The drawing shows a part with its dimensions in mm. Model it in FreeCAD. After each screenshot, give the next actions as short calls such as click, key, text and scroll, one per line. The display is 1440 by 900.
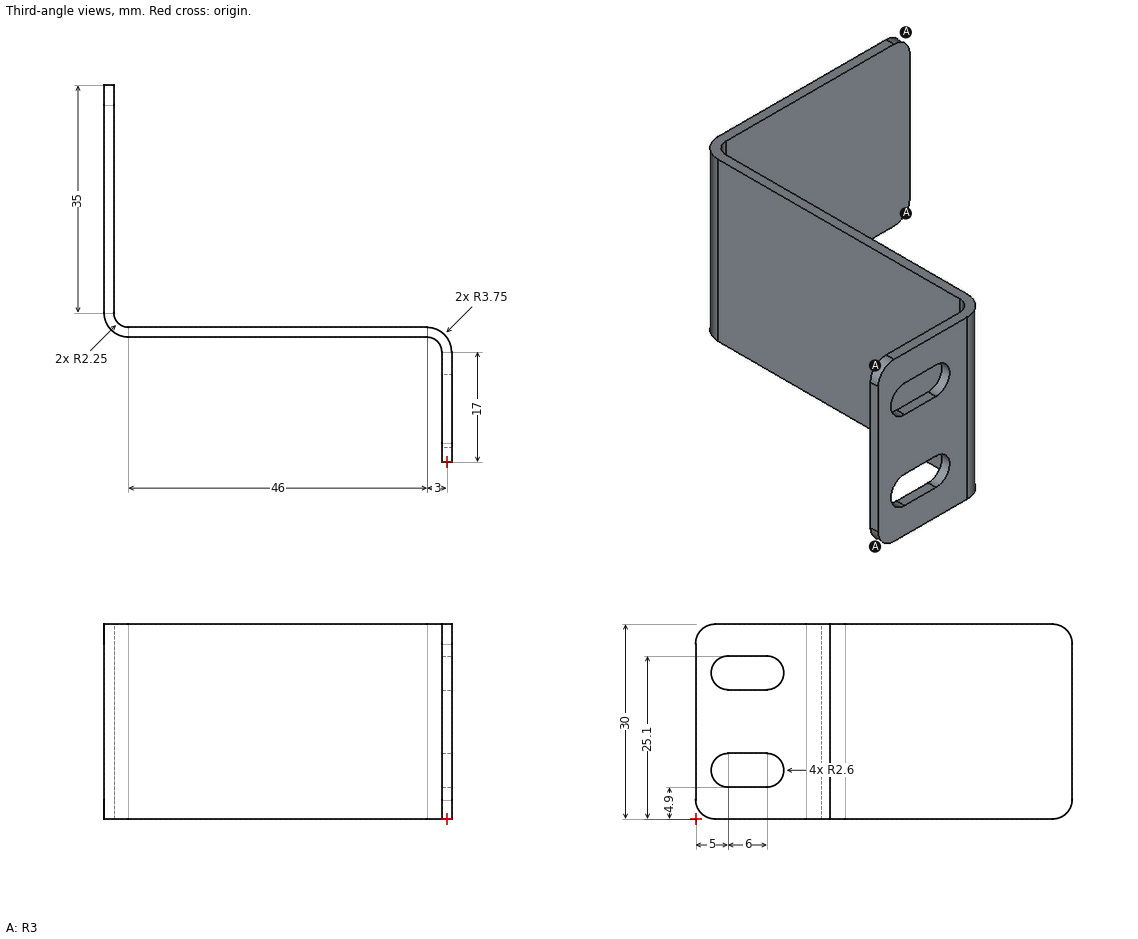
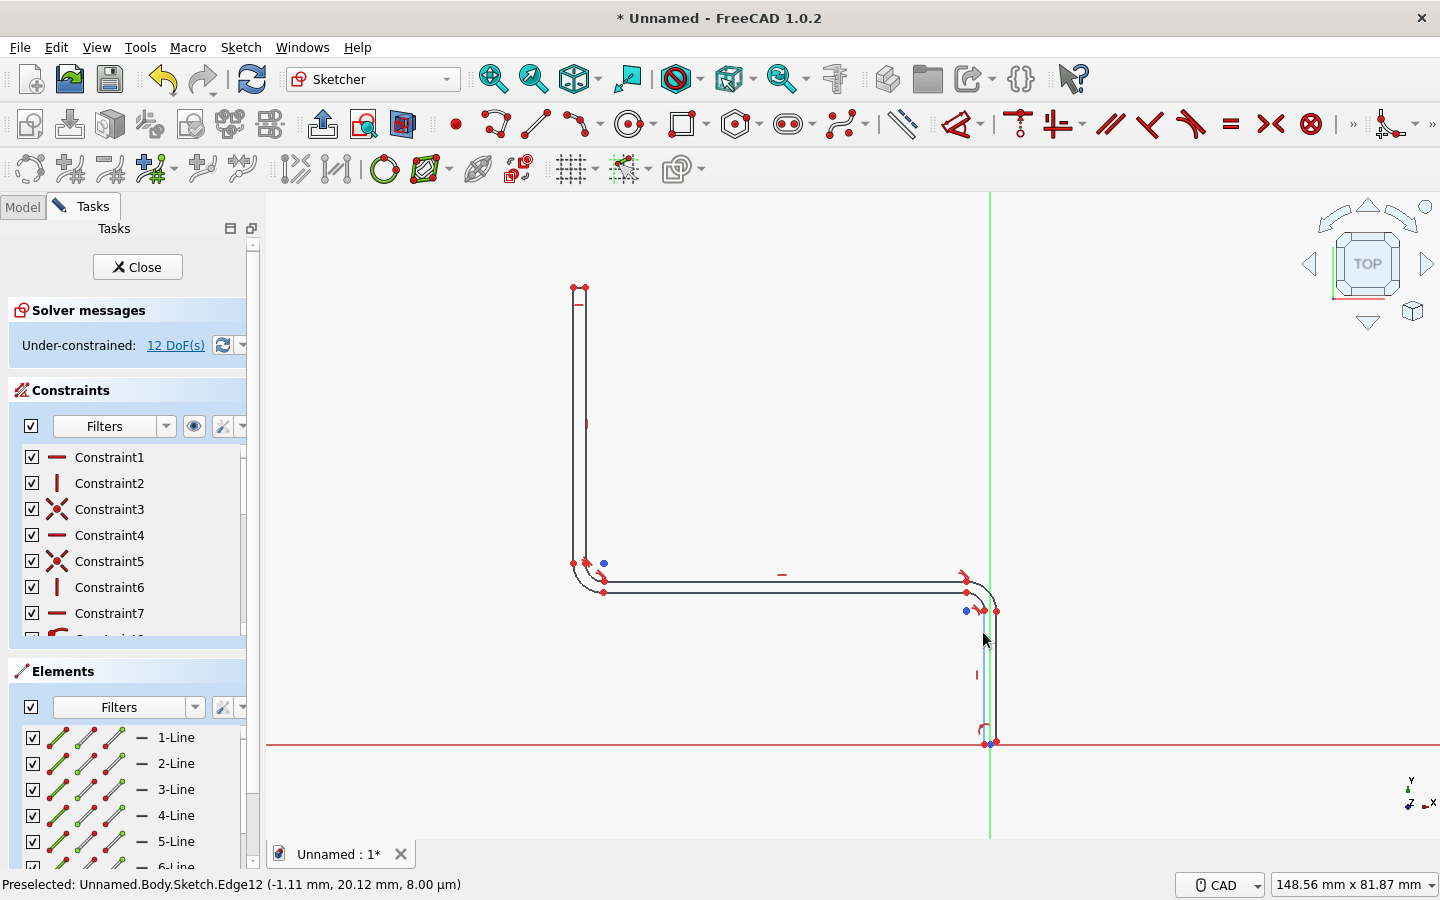
scroll(989, 744, up, 6)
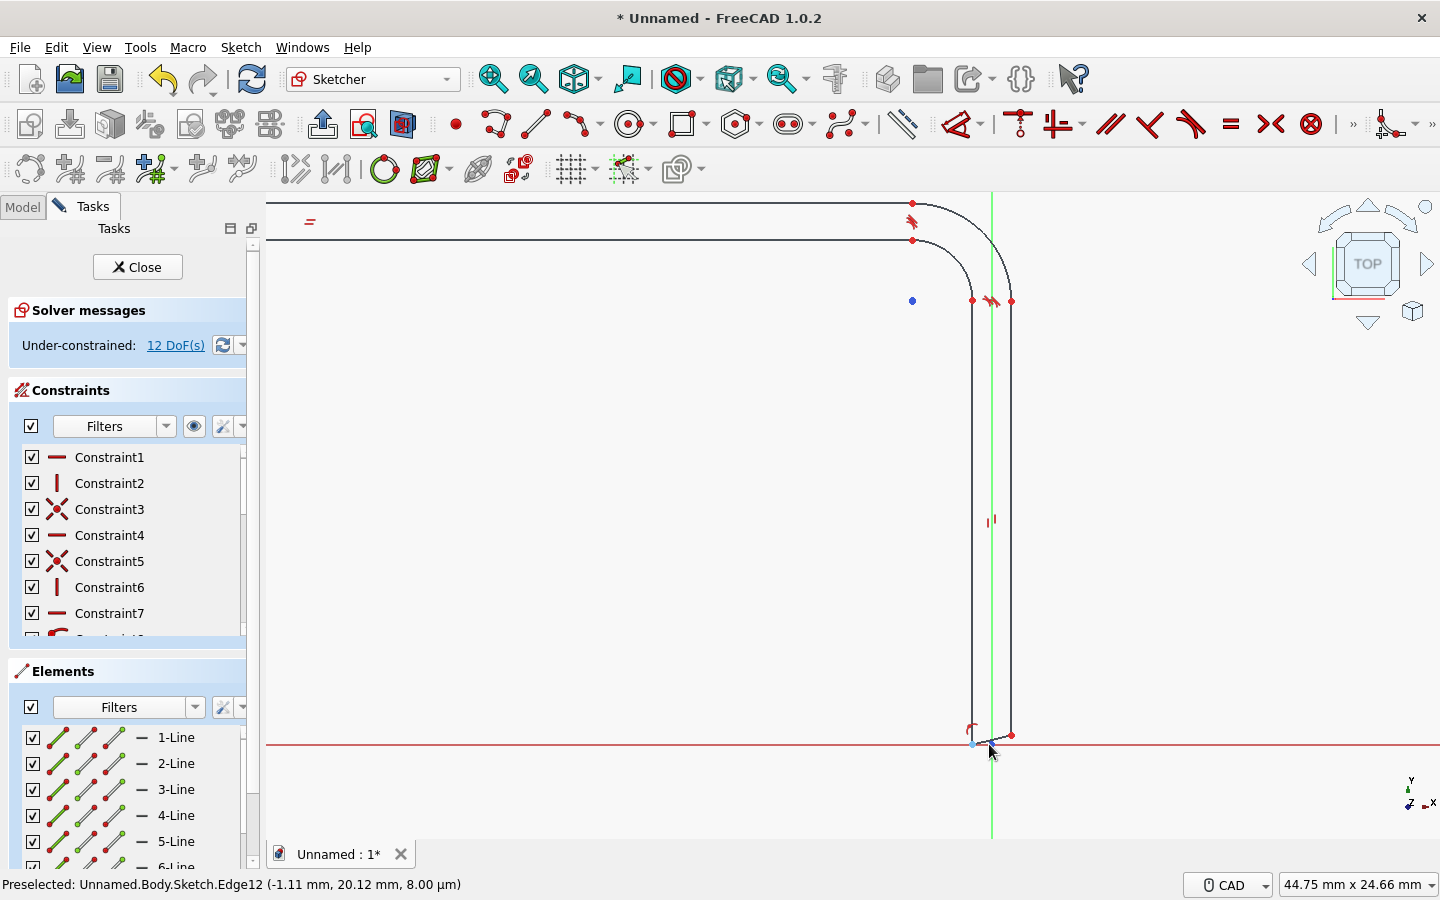
click(980, 743)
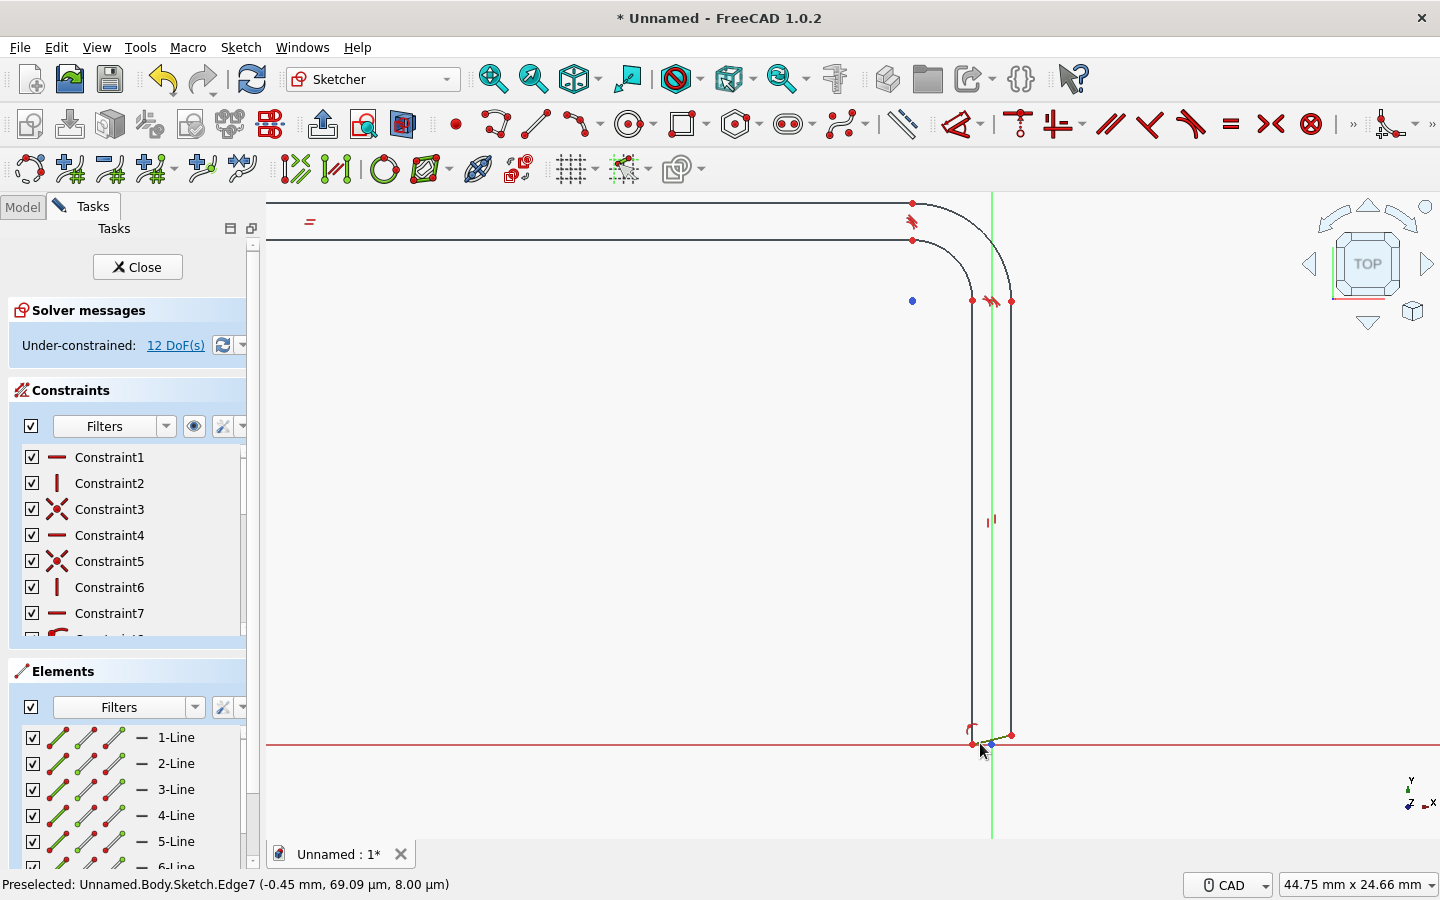
click(1084, 124)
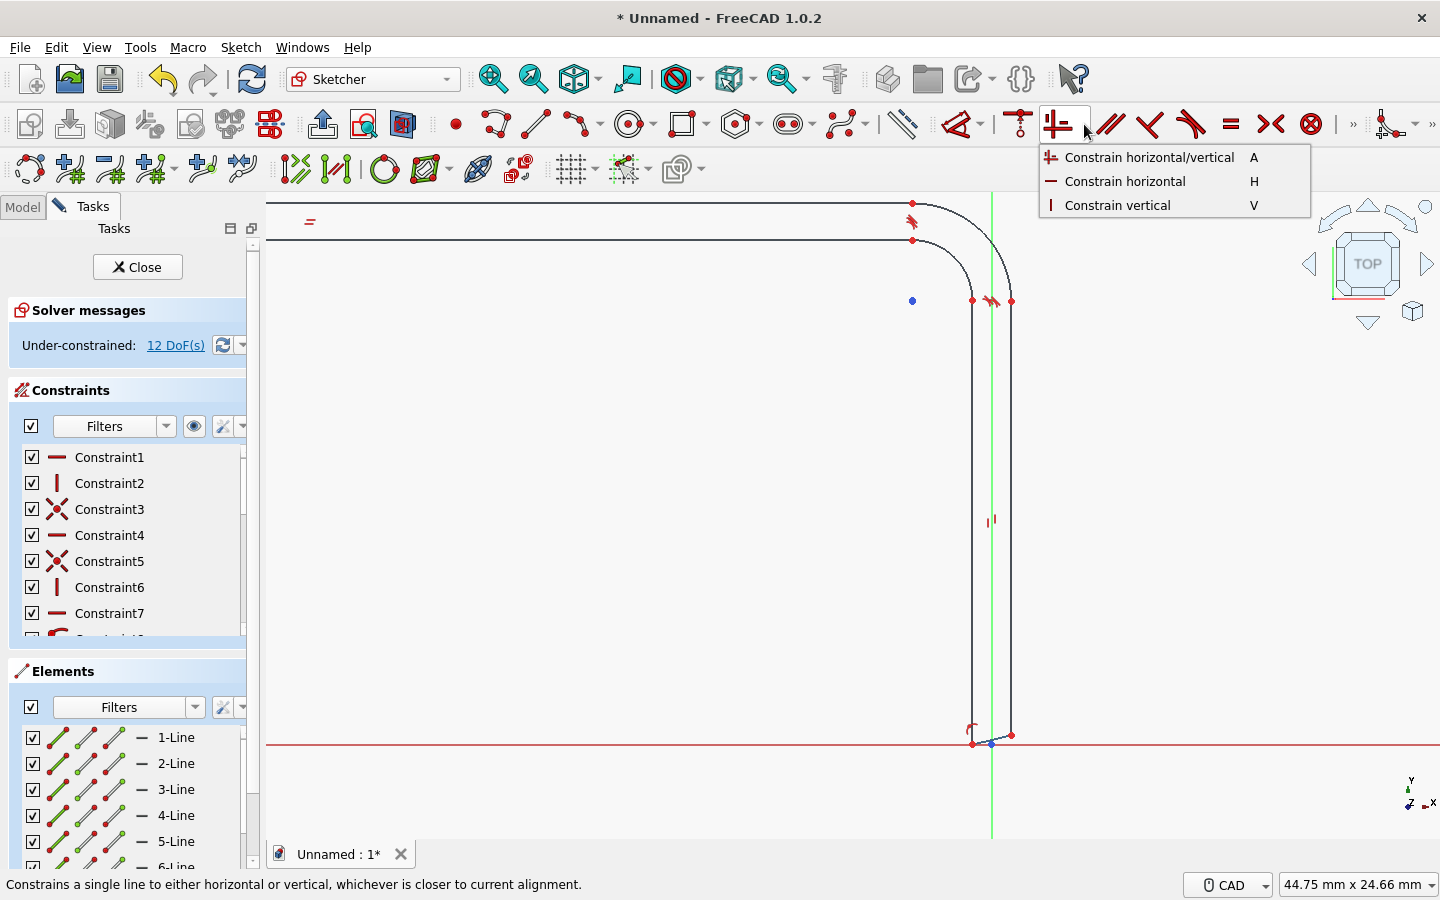
click(1175, 181)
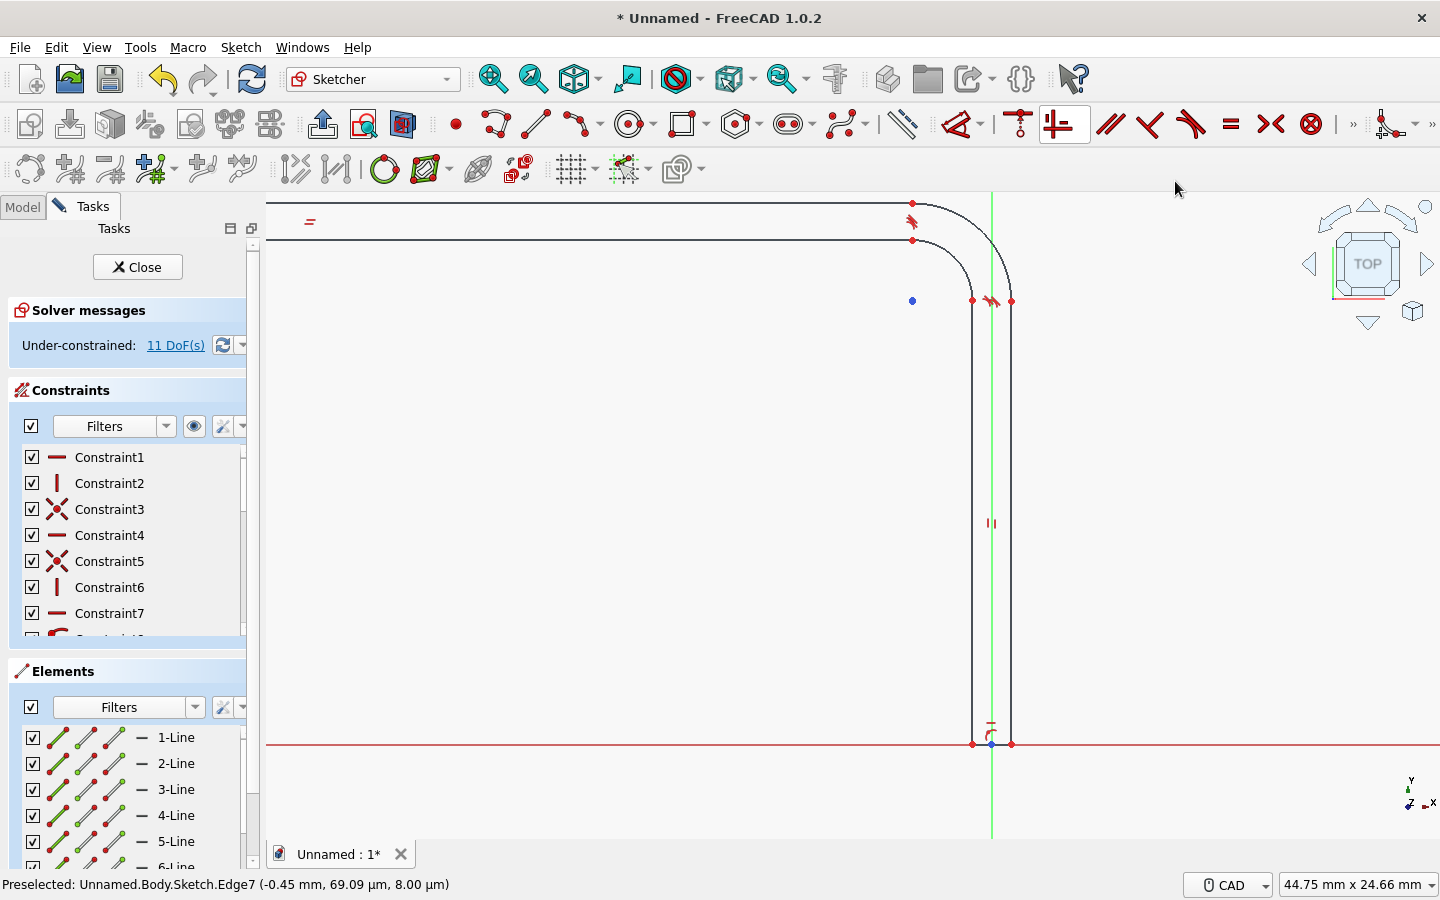
scroll(989, 745, down, 6)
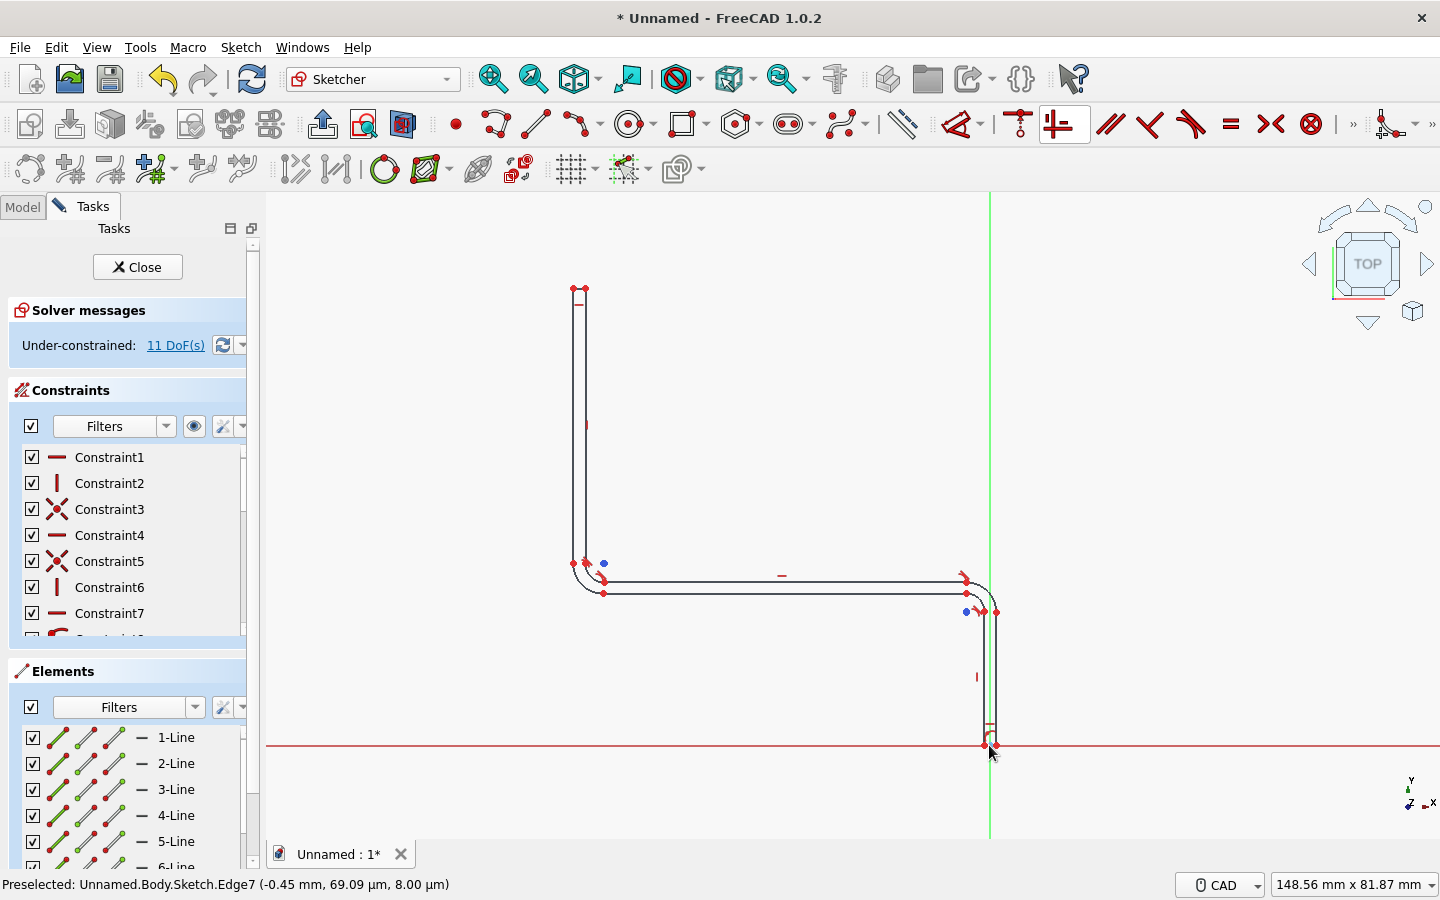
scroll(588, 572, up, 3)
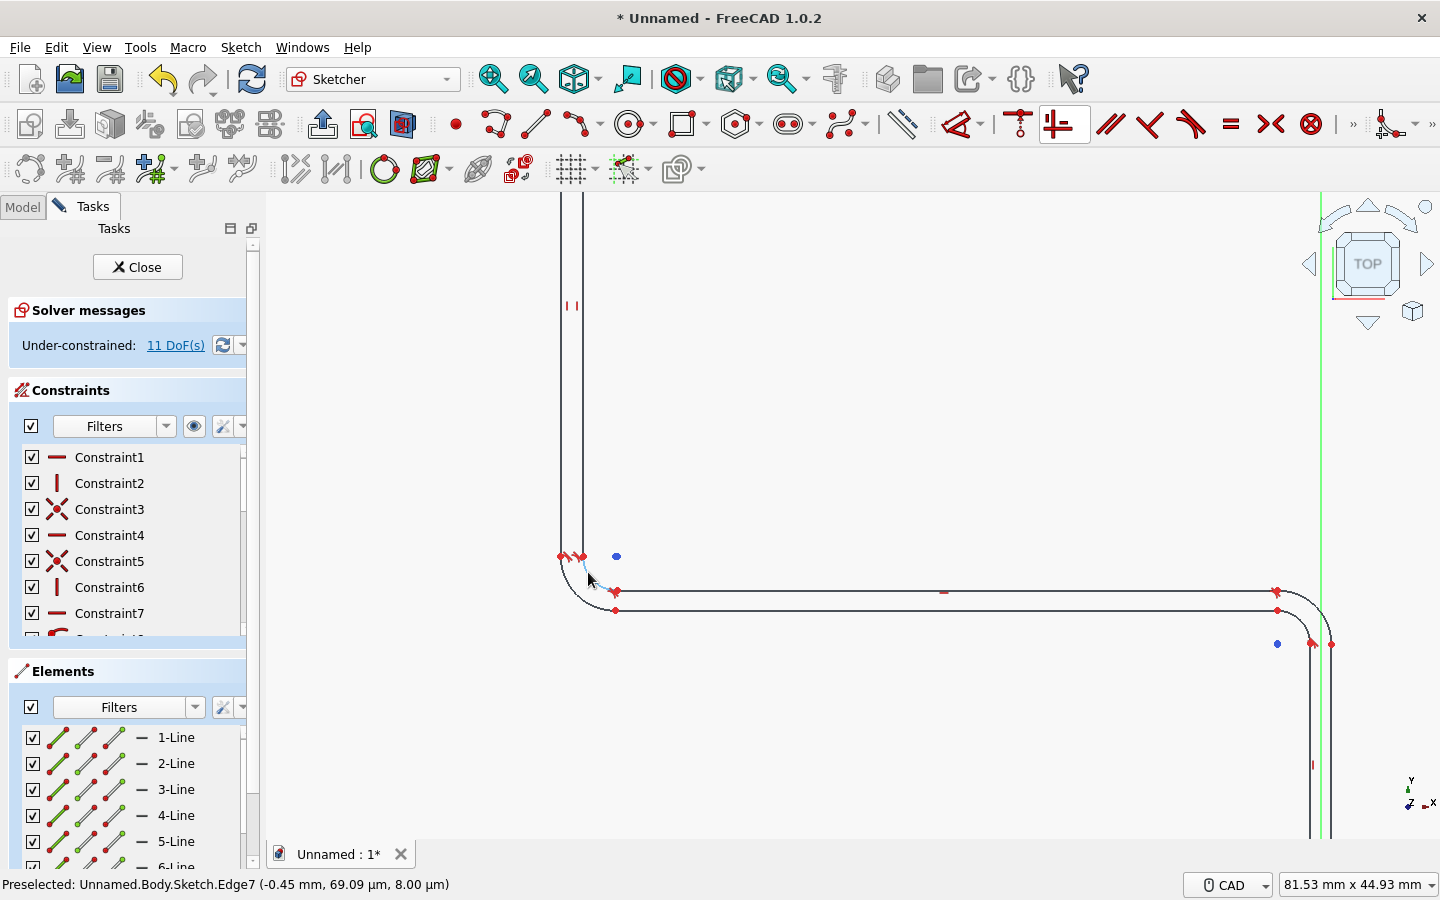
click(587, 572)